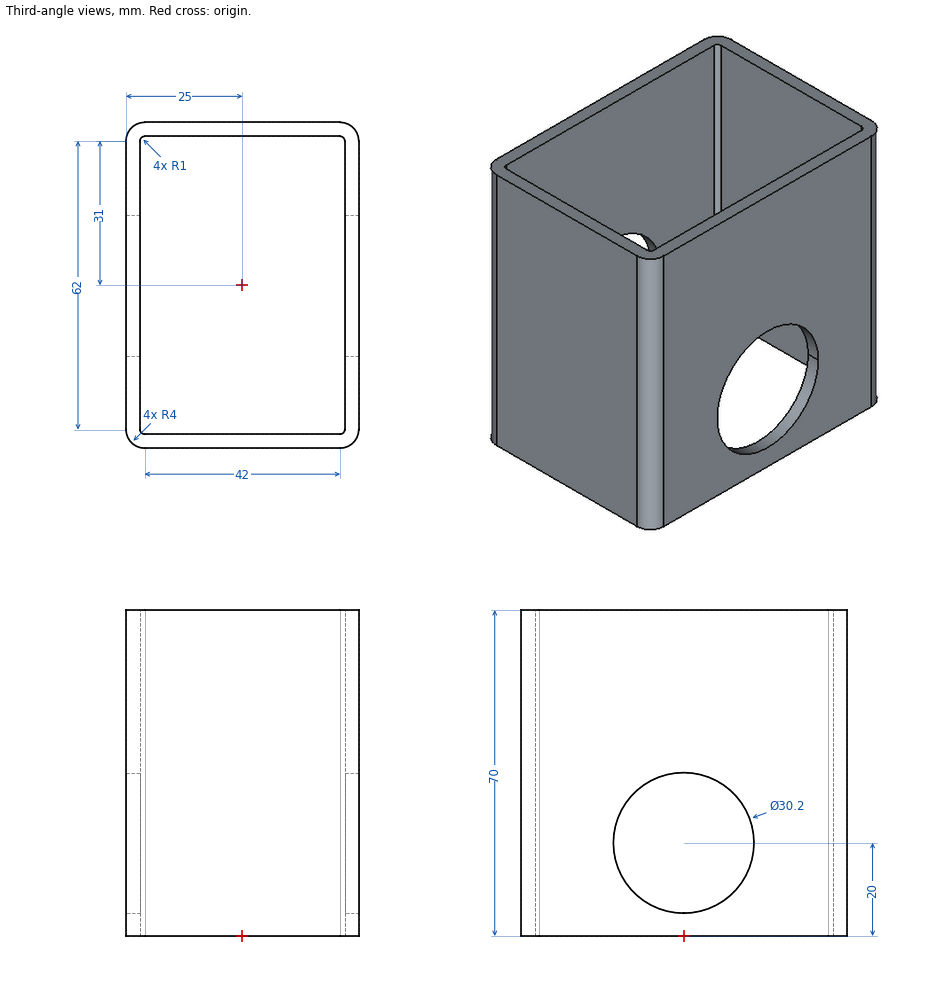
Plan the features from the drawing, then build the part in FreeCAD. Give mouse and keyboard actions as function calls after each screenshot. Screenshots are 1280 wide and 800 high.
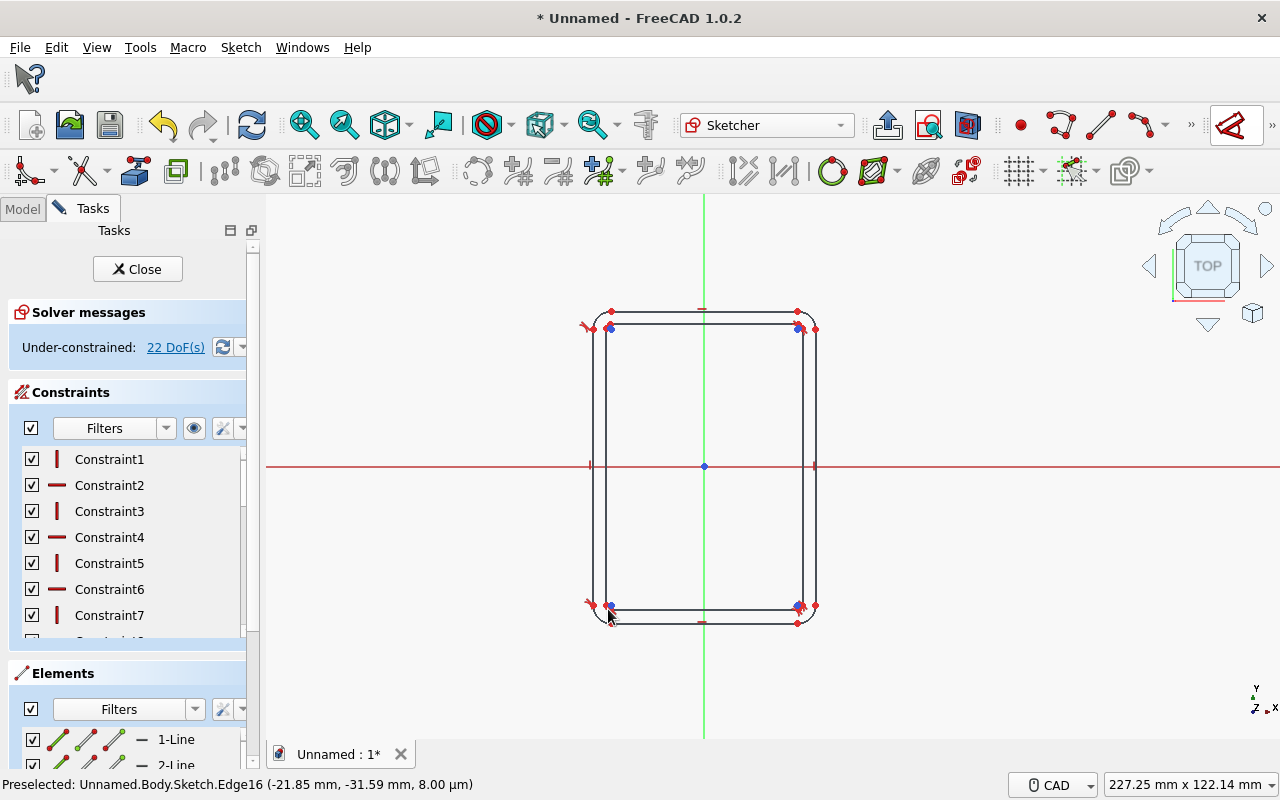
click(667, 324)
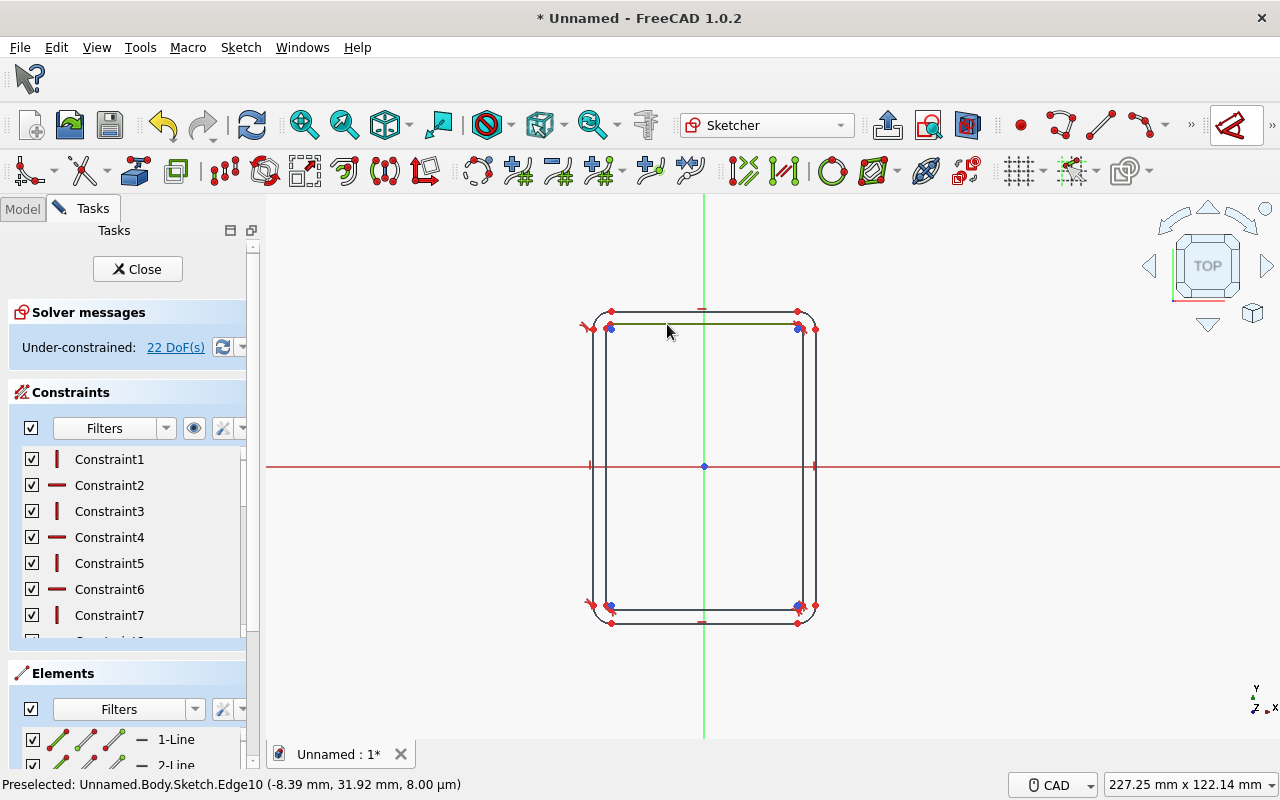
scroll(607, 326, up, 7)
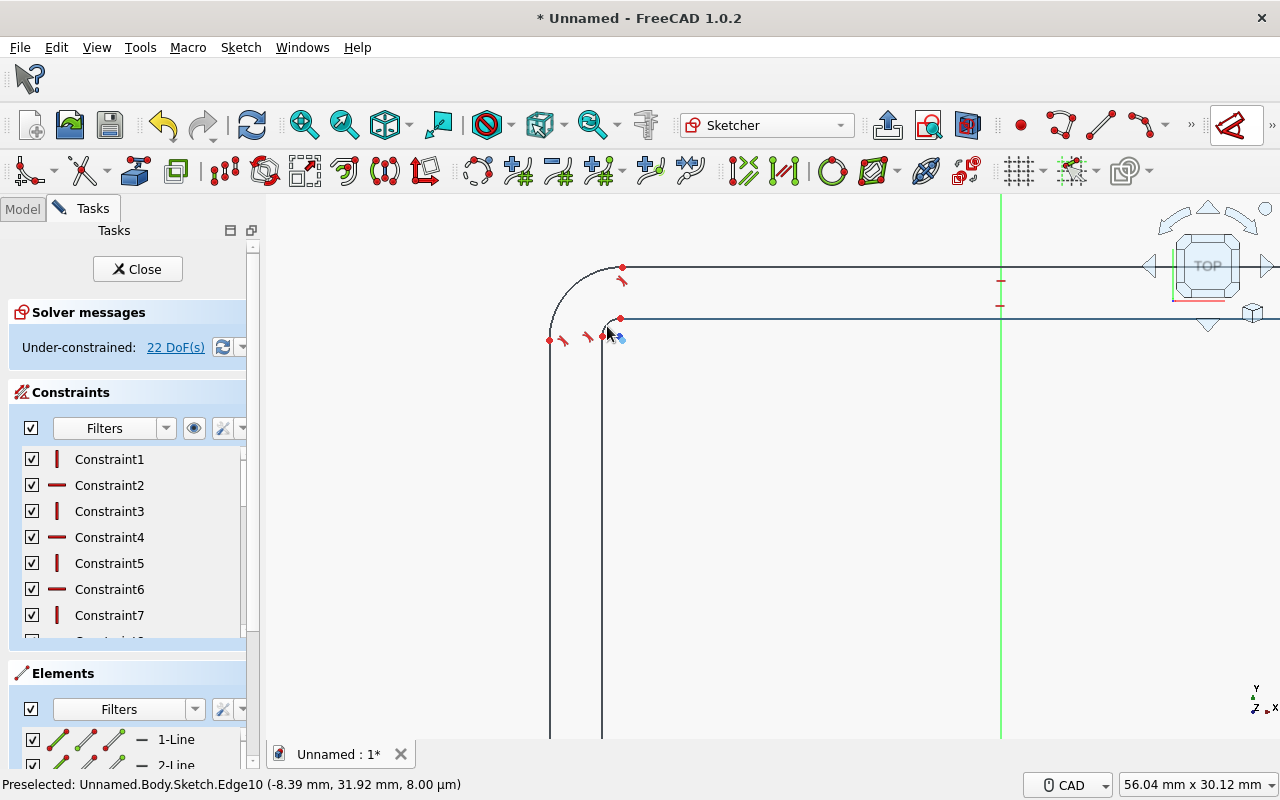
click(608, 324)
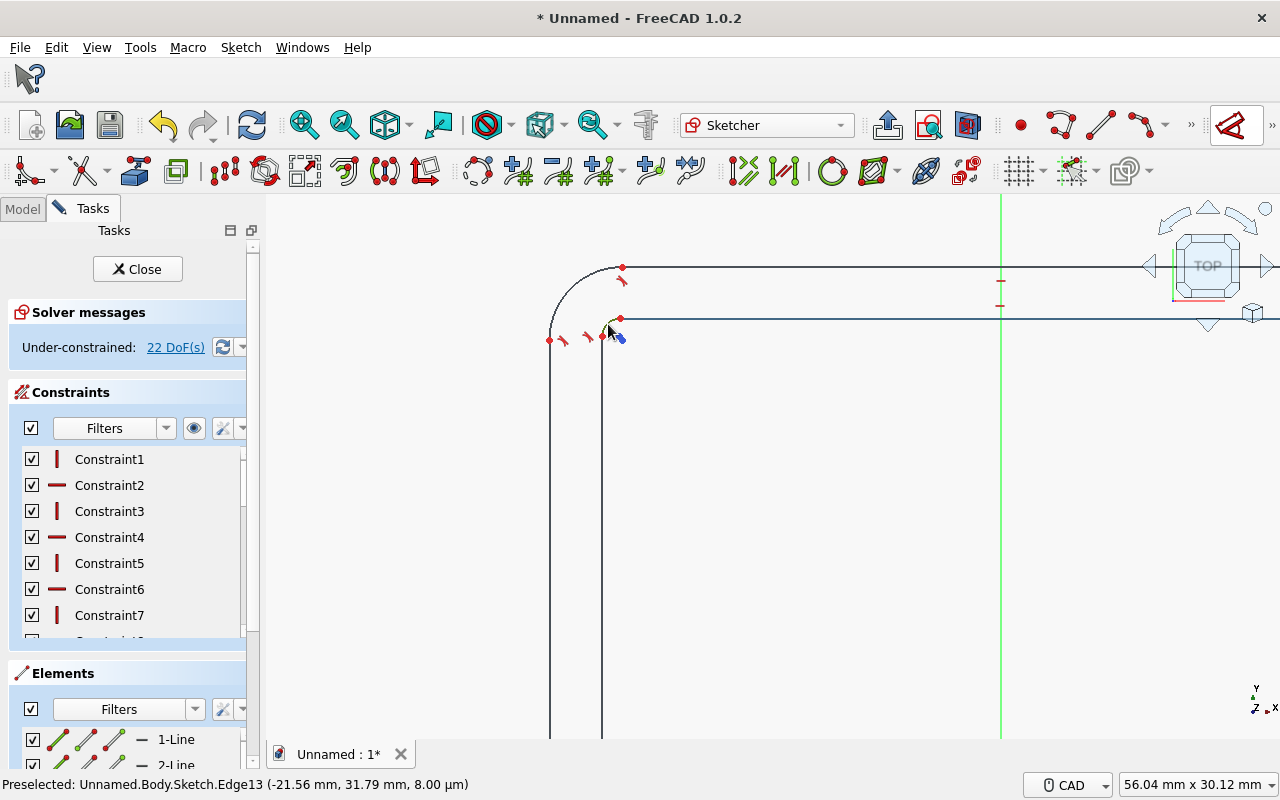
key(t)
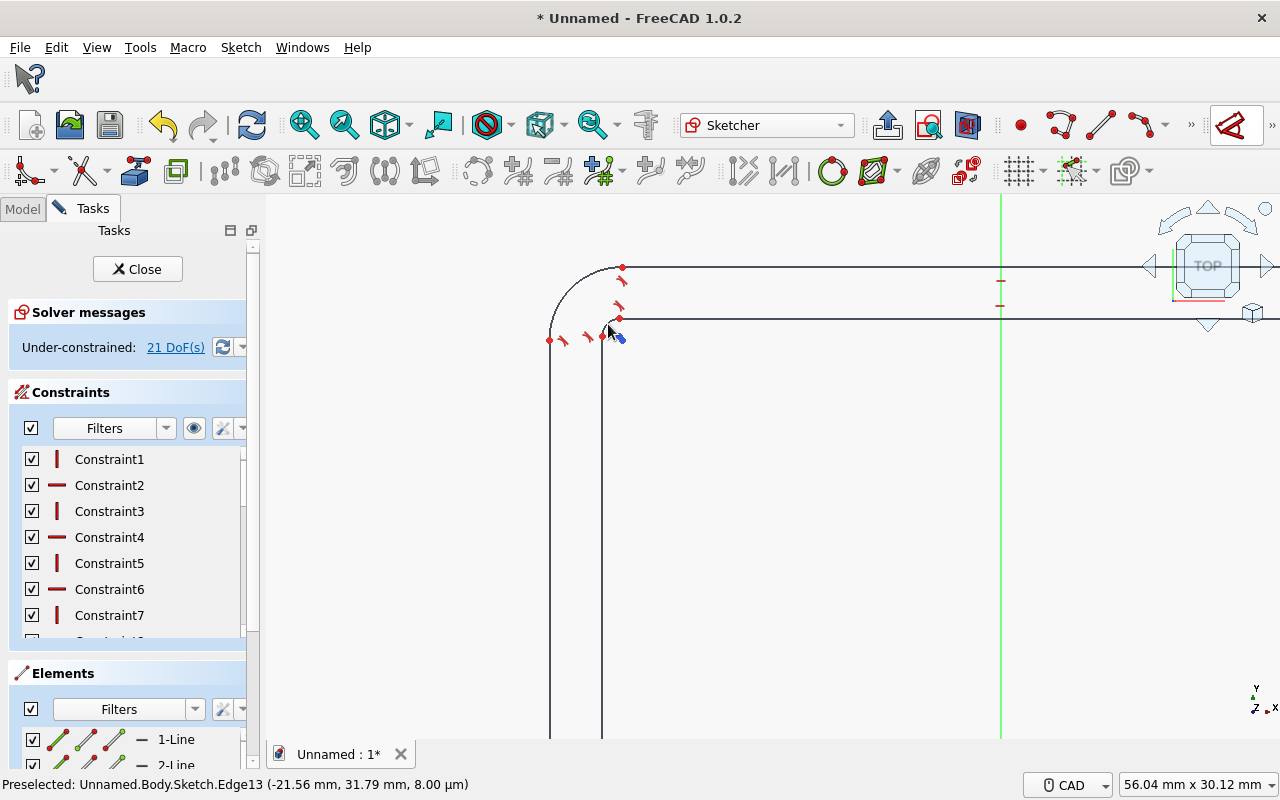
click(848, 319)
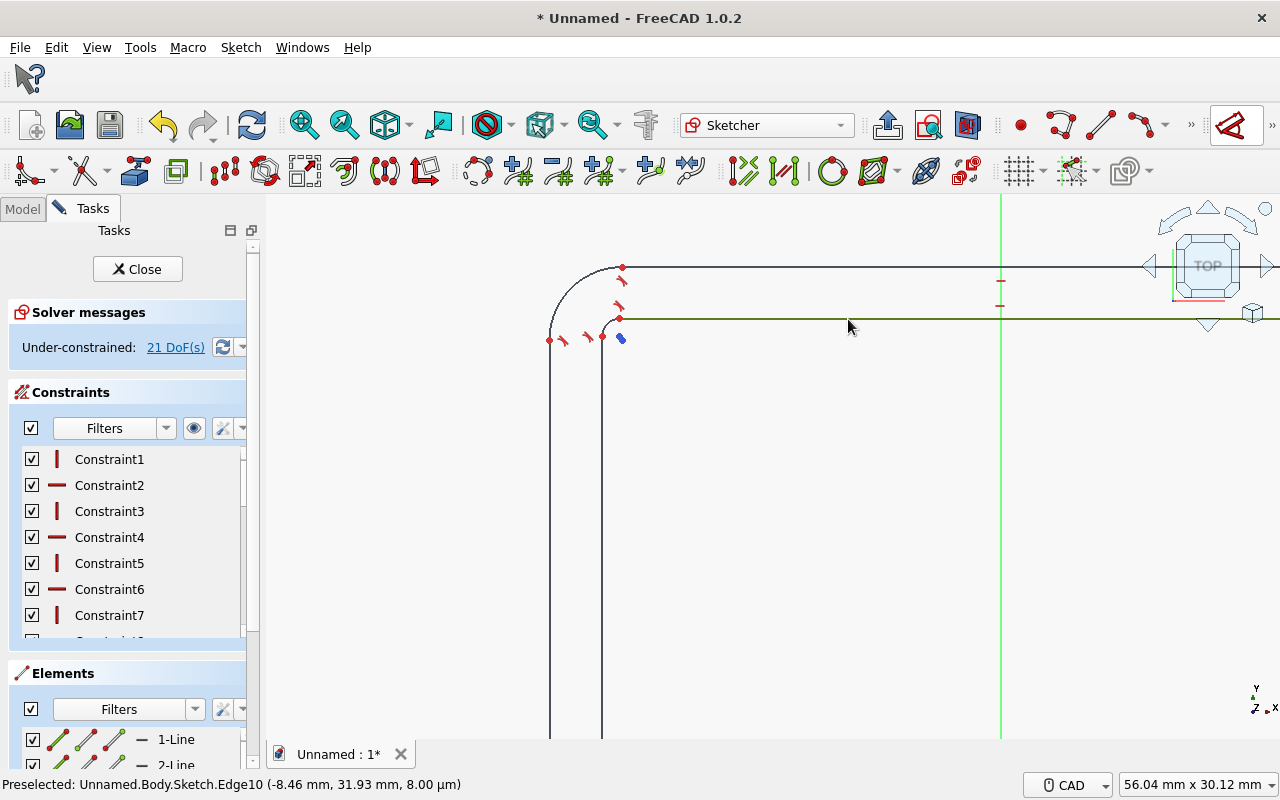
scroll(607, 326, down, 7)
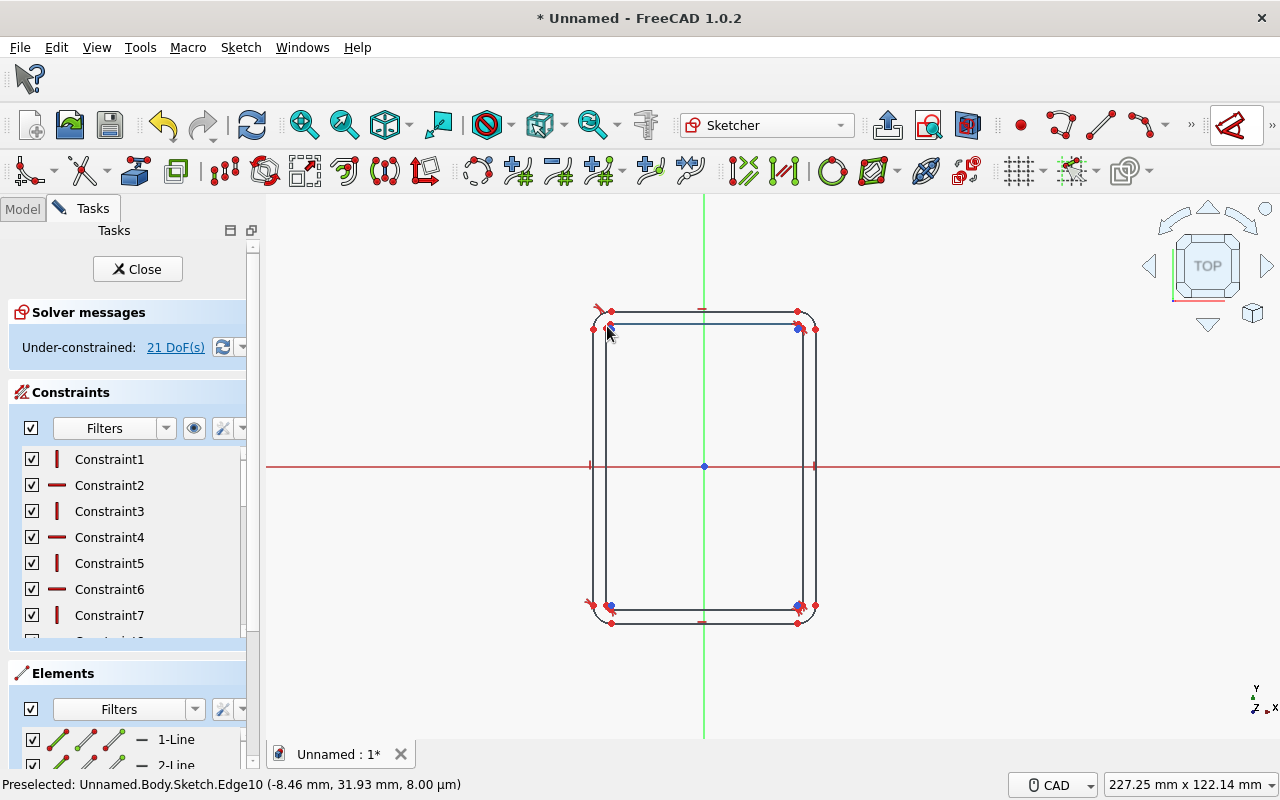
scroll(801, 326, up, 7)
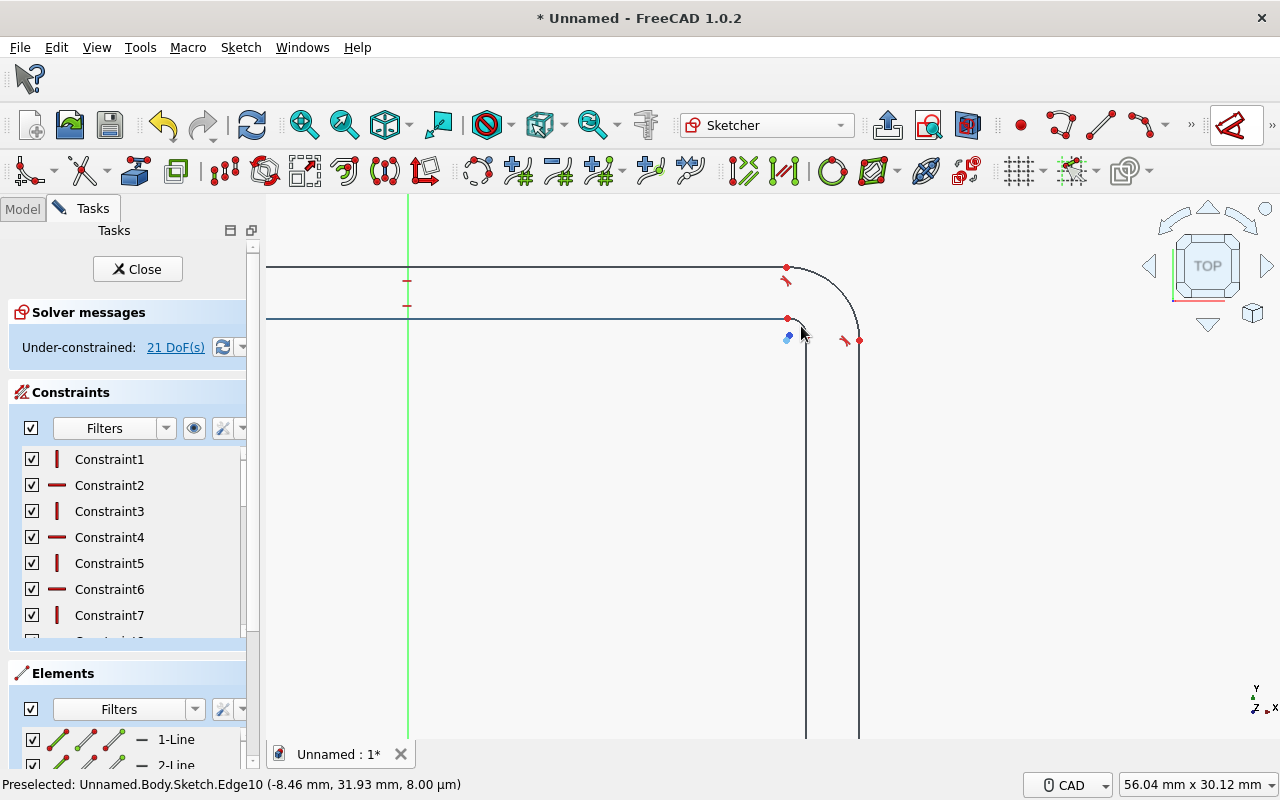
click(801, 323)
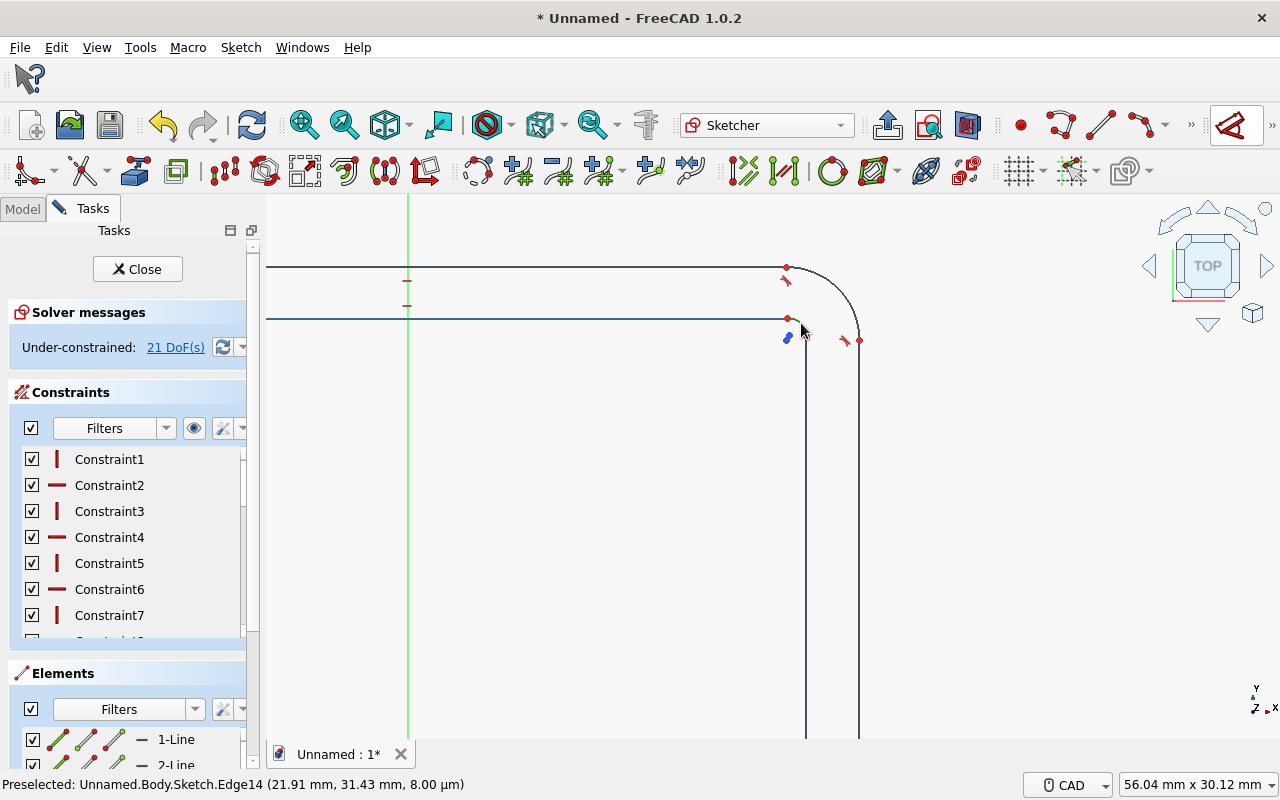
key(t)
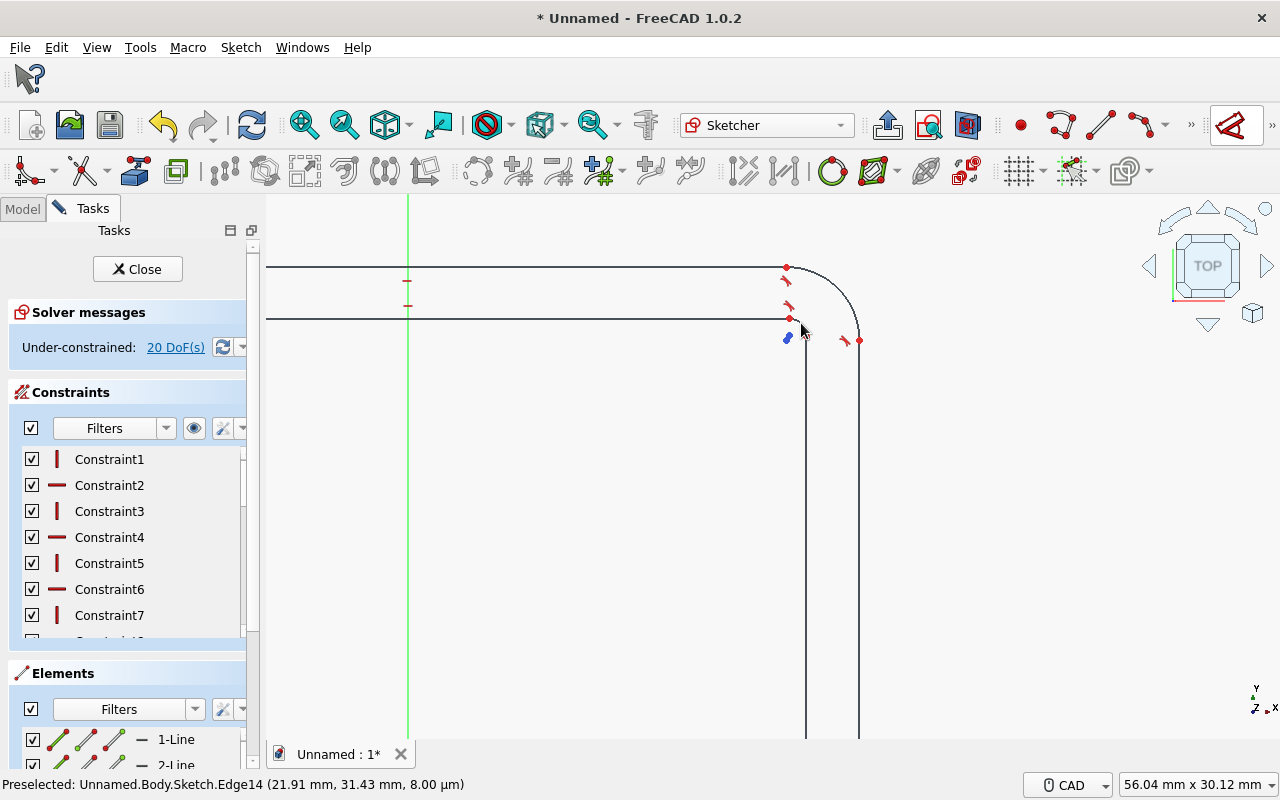
click(806, 673)